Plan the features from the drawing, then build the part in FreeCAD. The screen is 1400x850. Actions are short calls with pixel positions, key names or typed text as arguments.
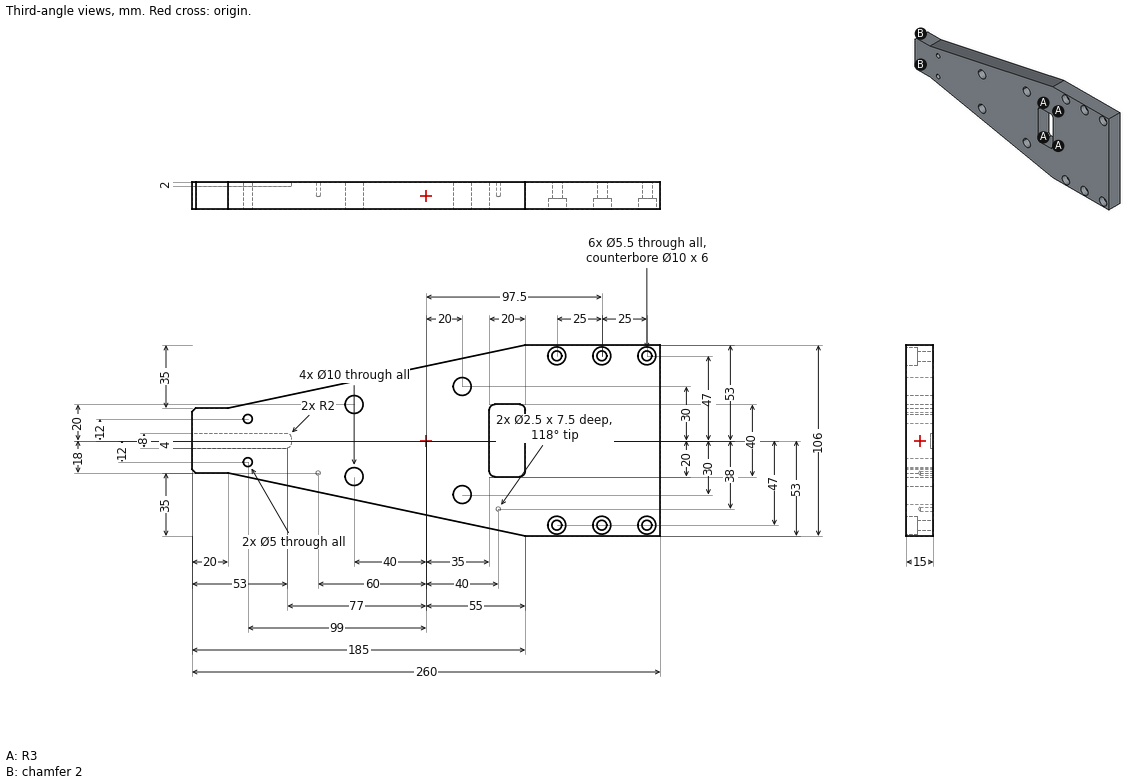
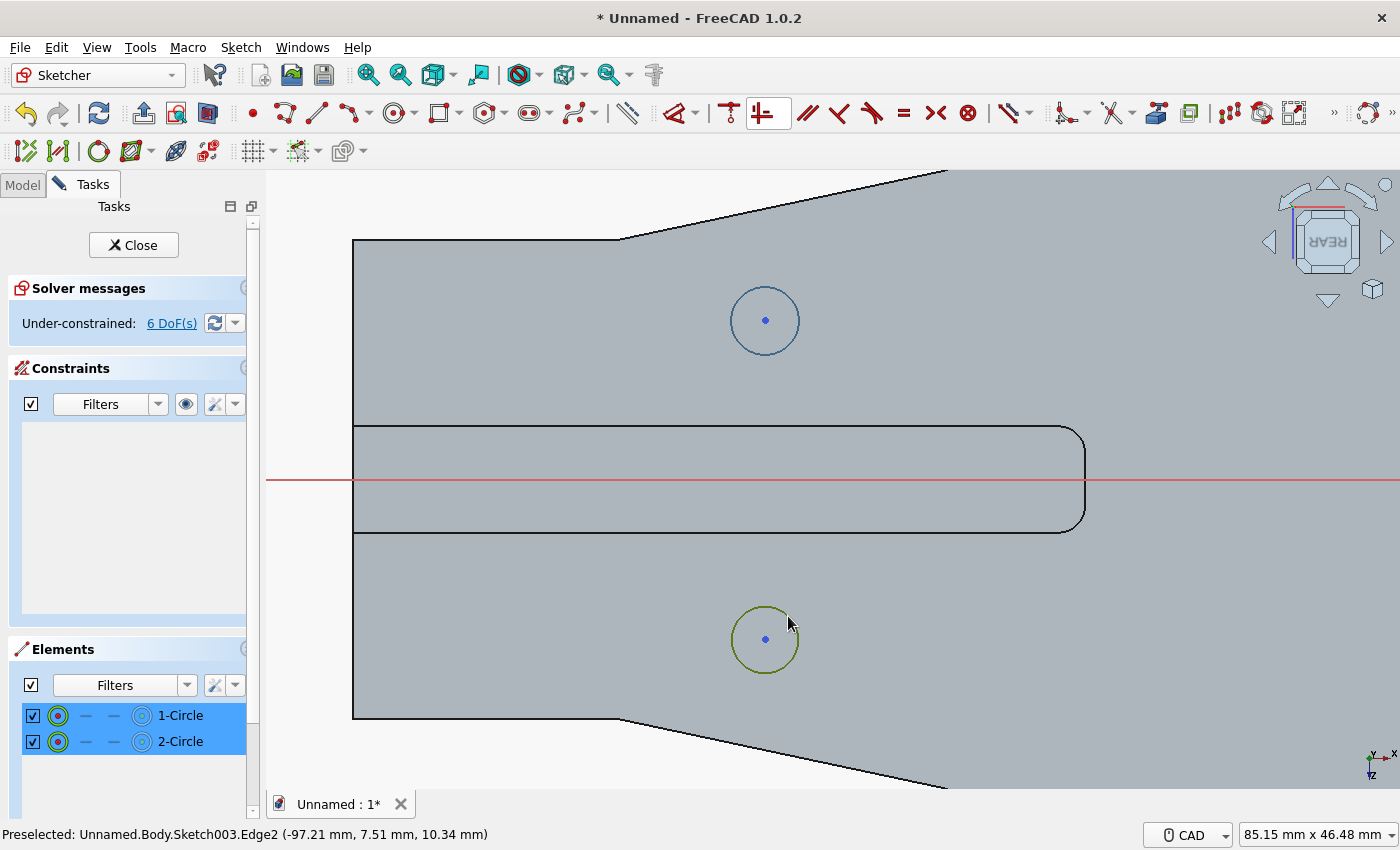
key(e)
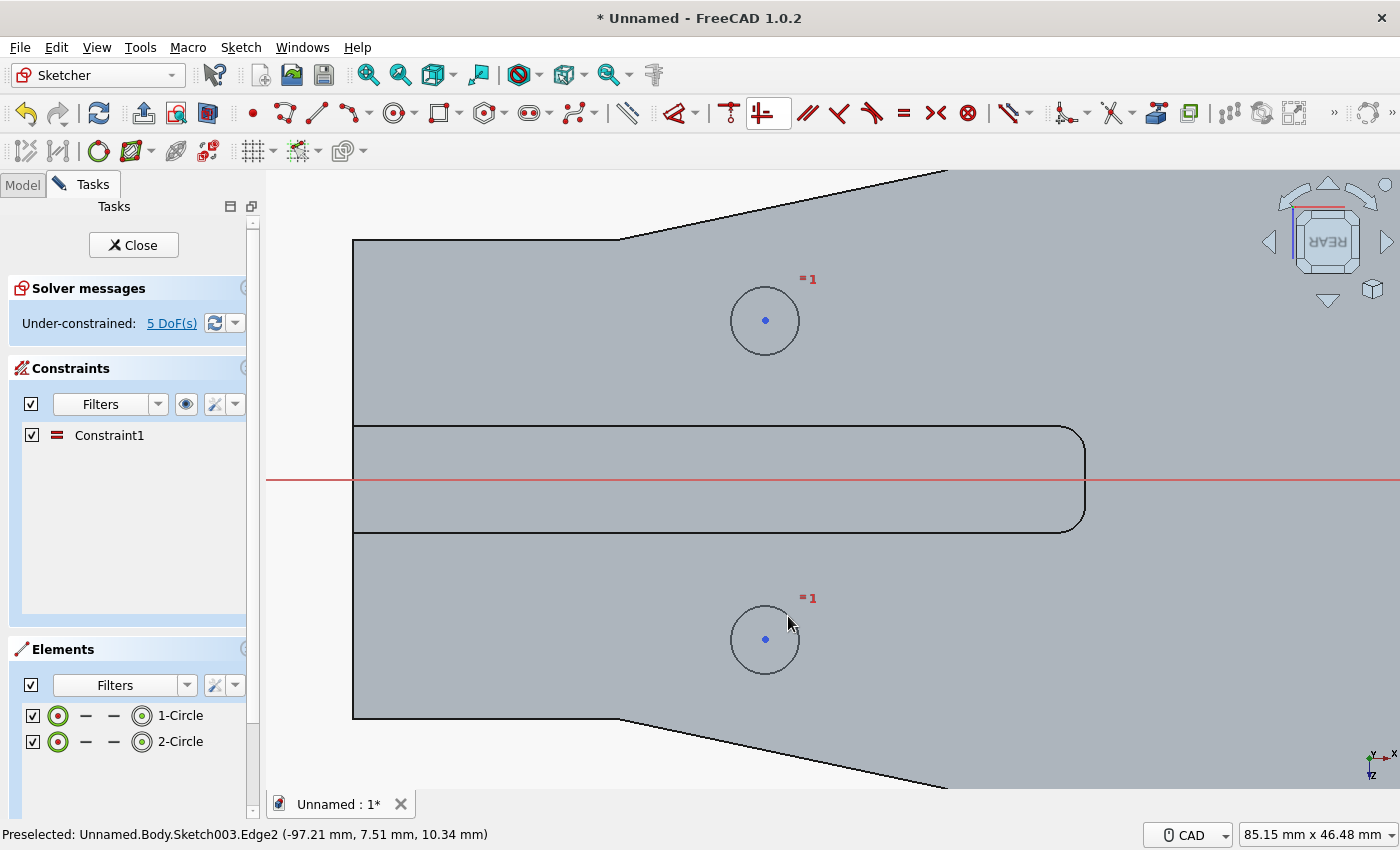
click(765, 321)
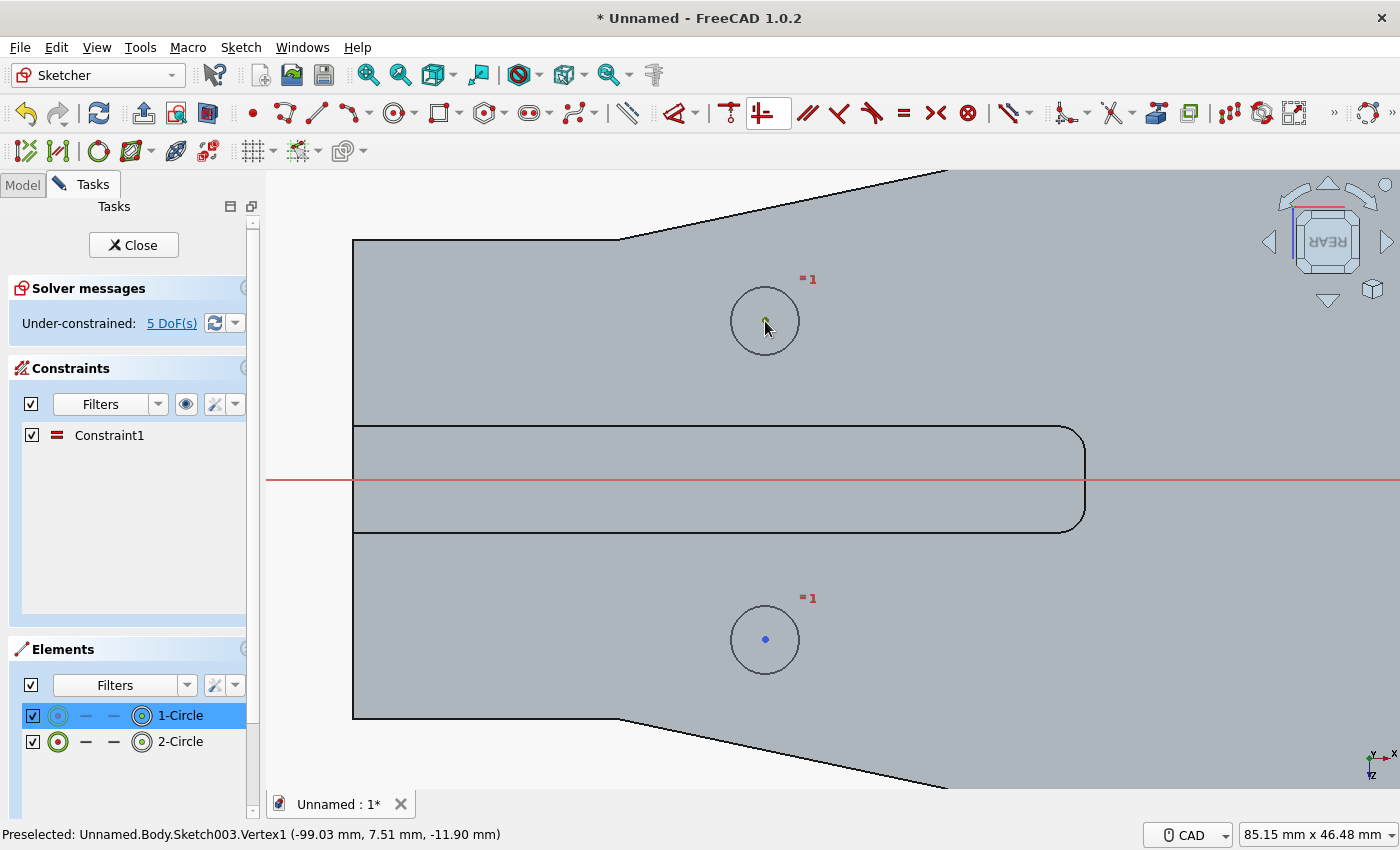
click(765, 640)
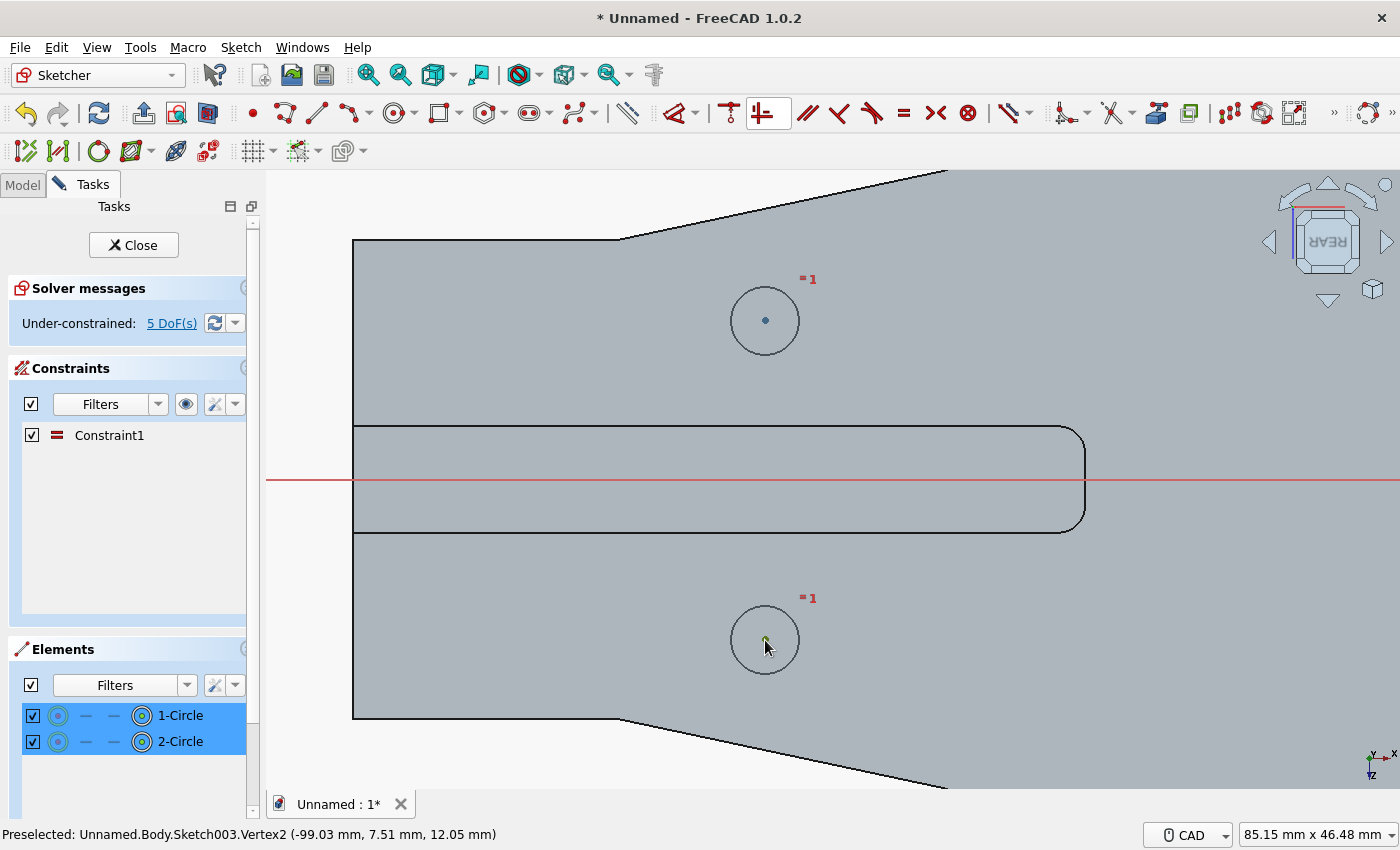
key(v)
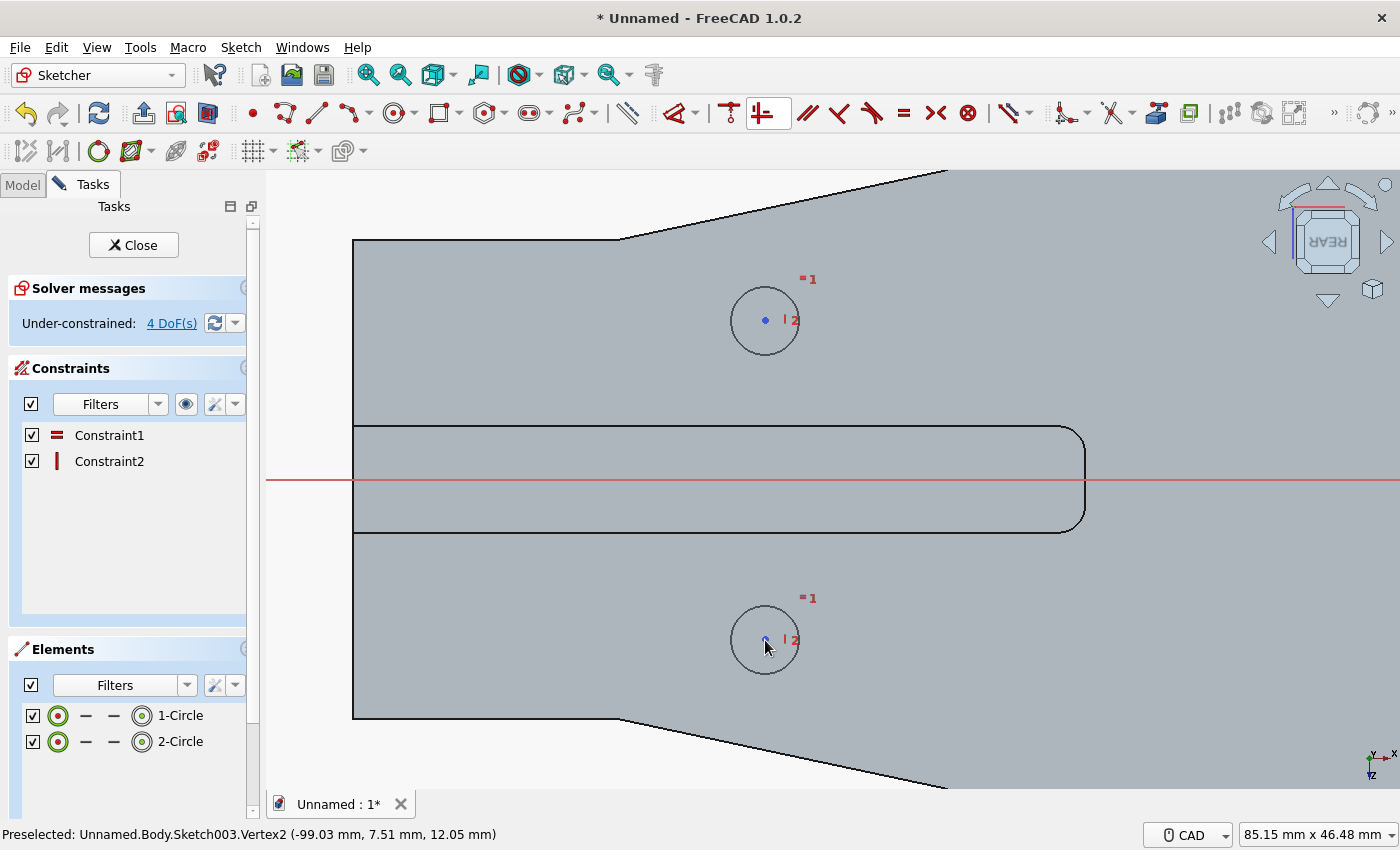
key(d)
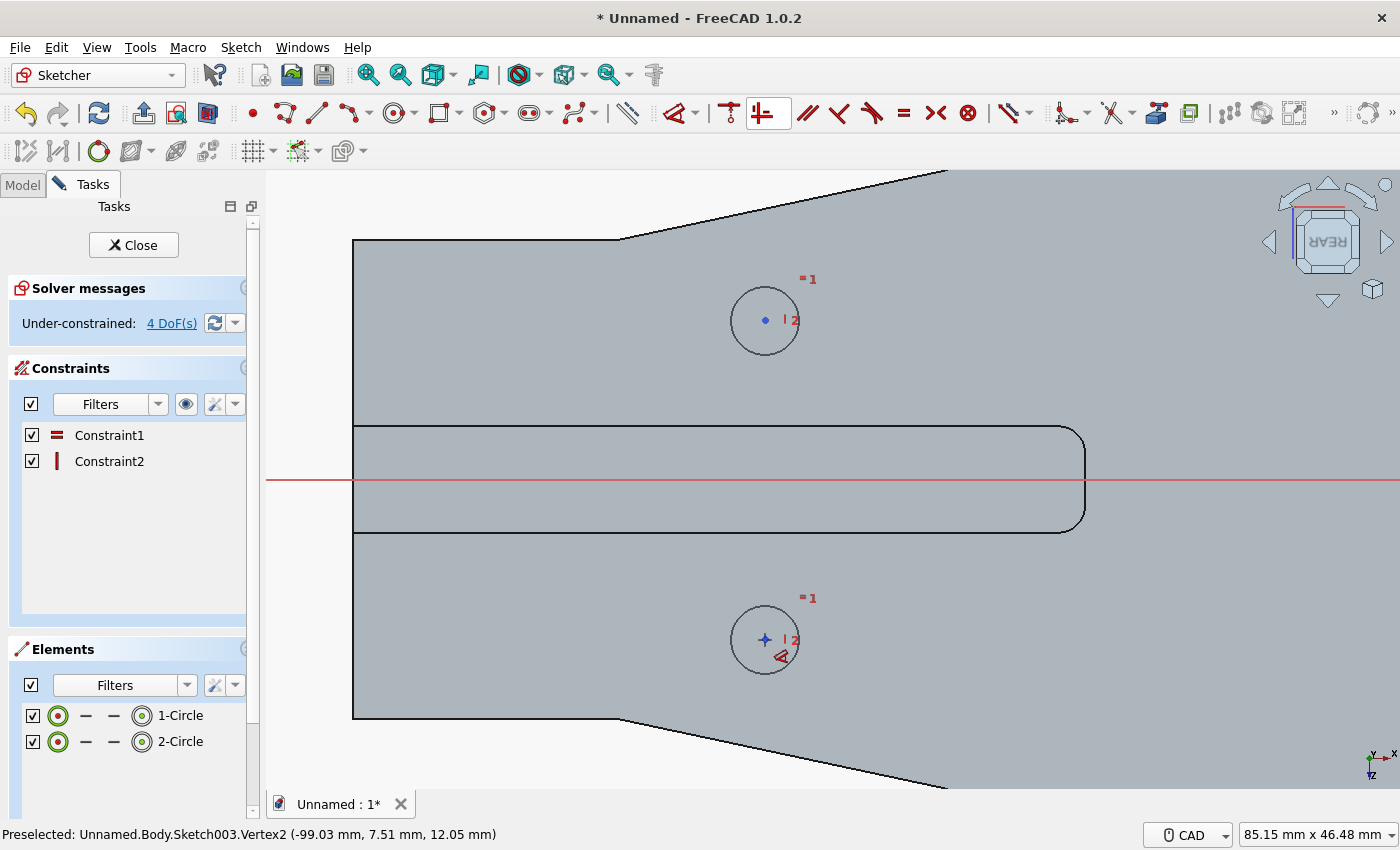
click(789, 297)
click(812, 274)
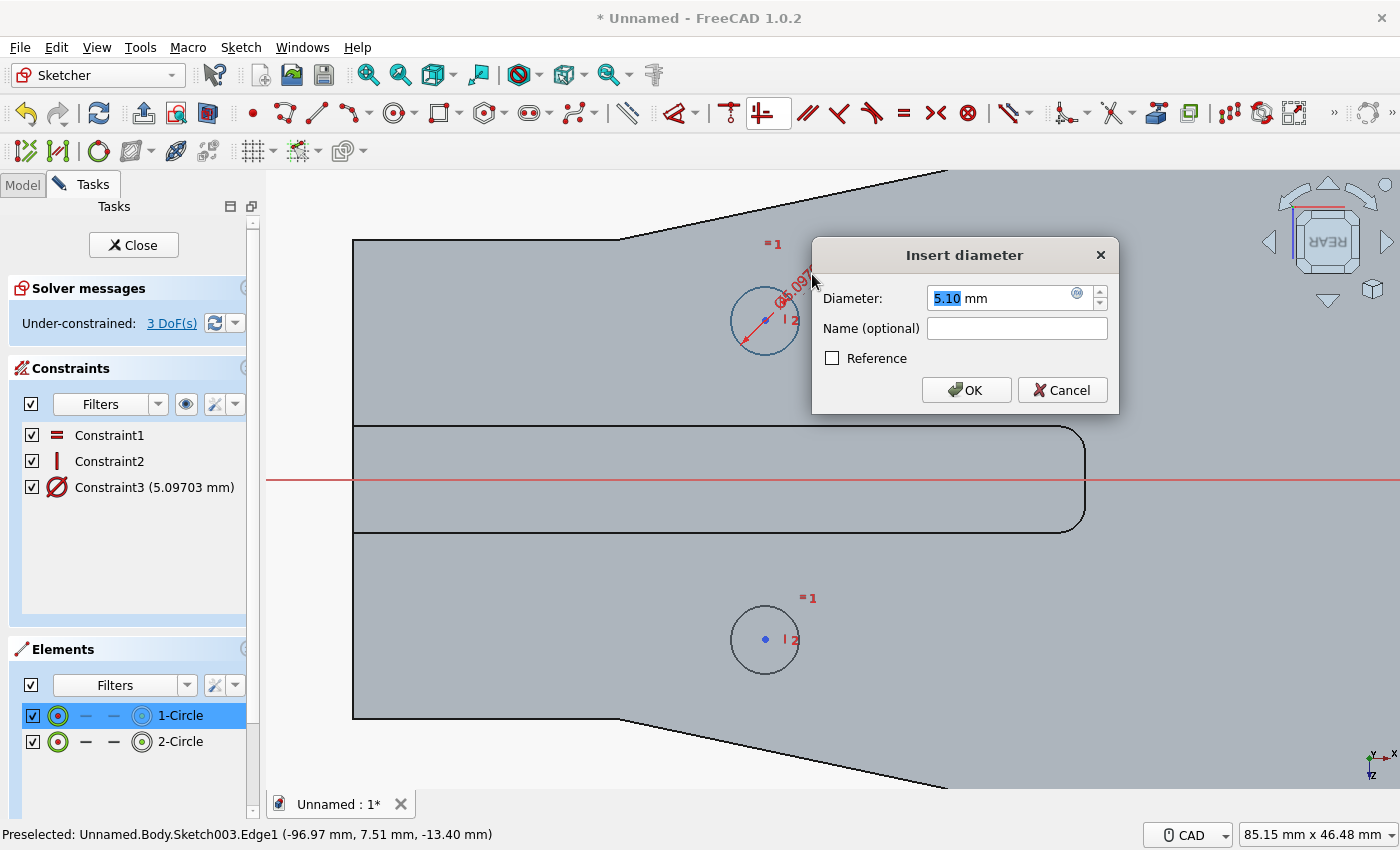
text(5)
key(Return)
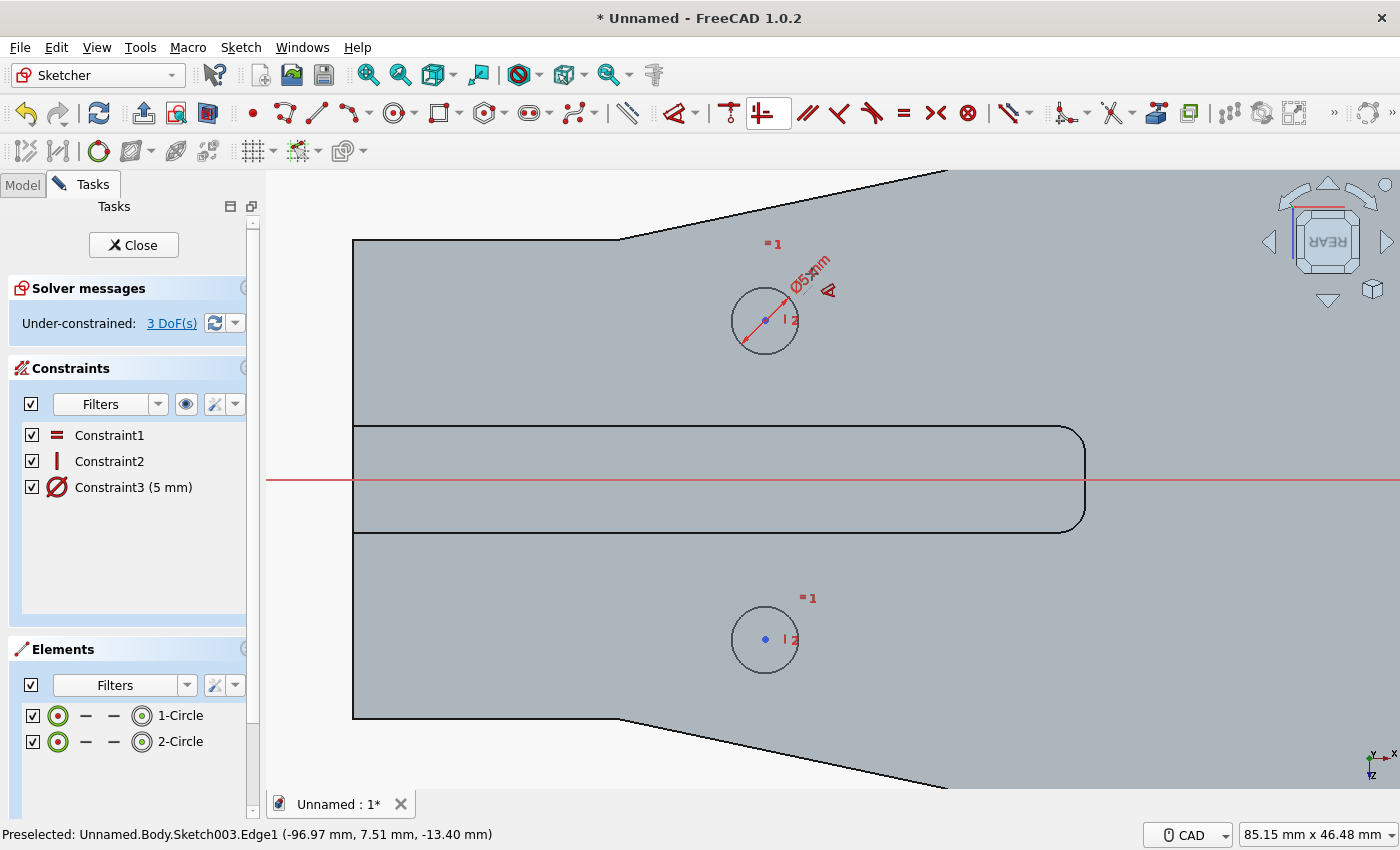
click(765, 321)
click(1000, 287)